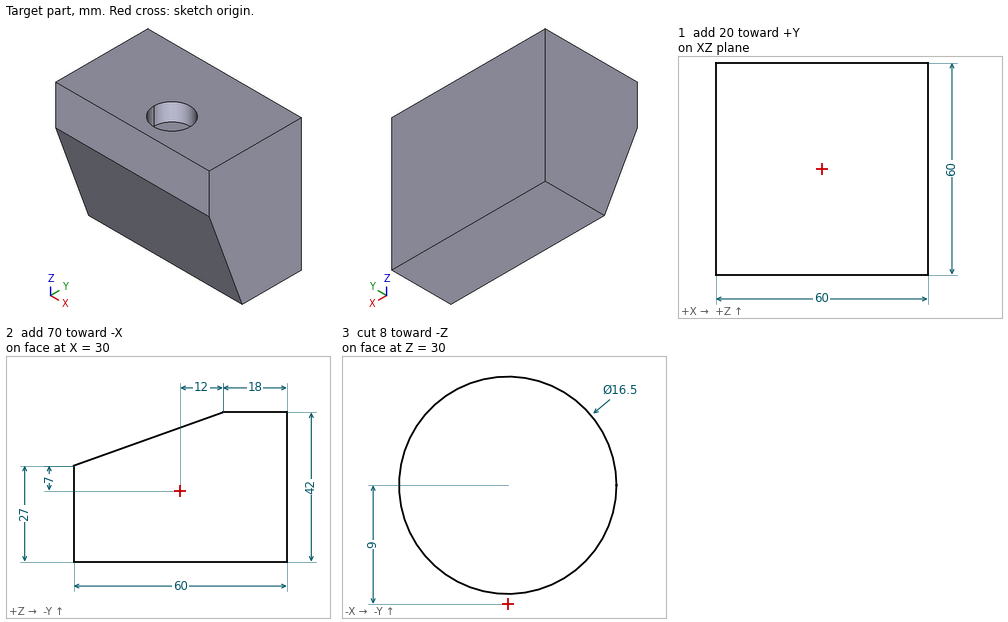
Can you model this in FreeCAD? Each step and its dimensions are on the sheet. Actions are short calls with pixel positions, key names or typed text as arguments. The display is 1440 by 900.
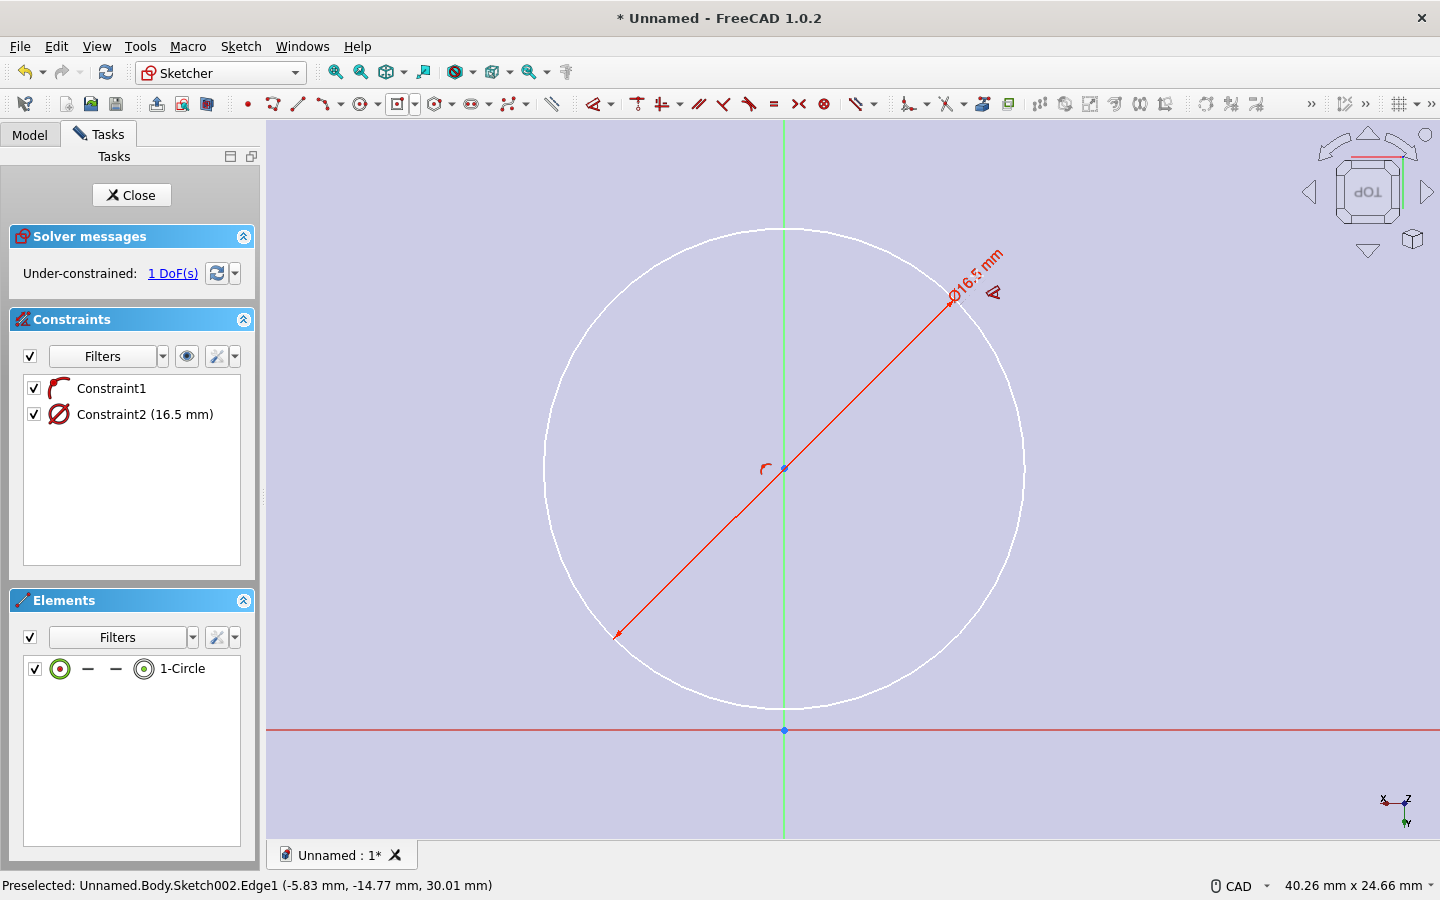
click(784, 469)
click(818, 600)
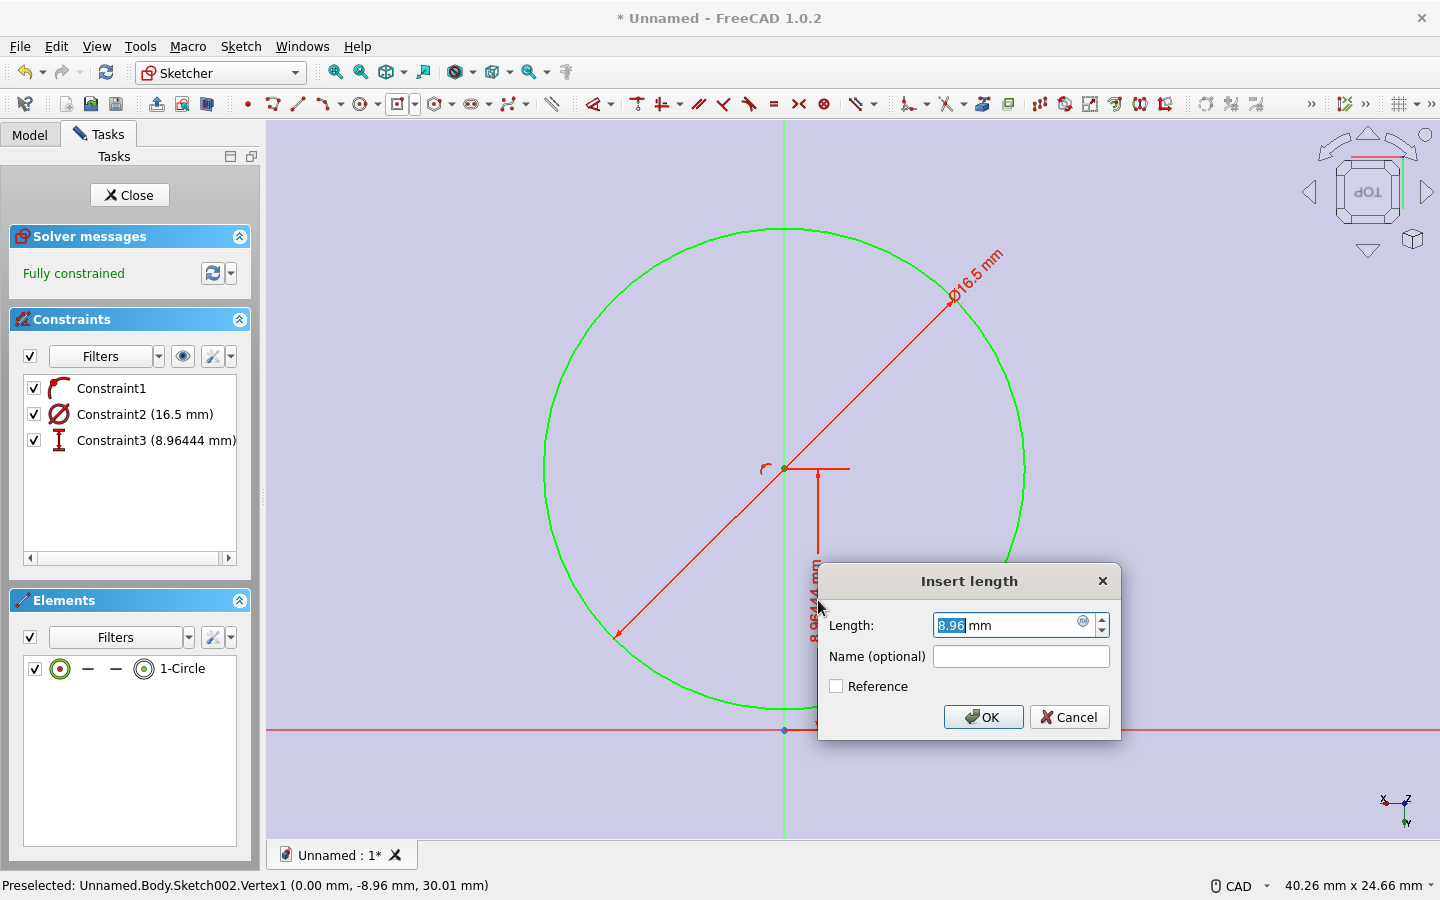
text(9)
key(Return)
key(Escape)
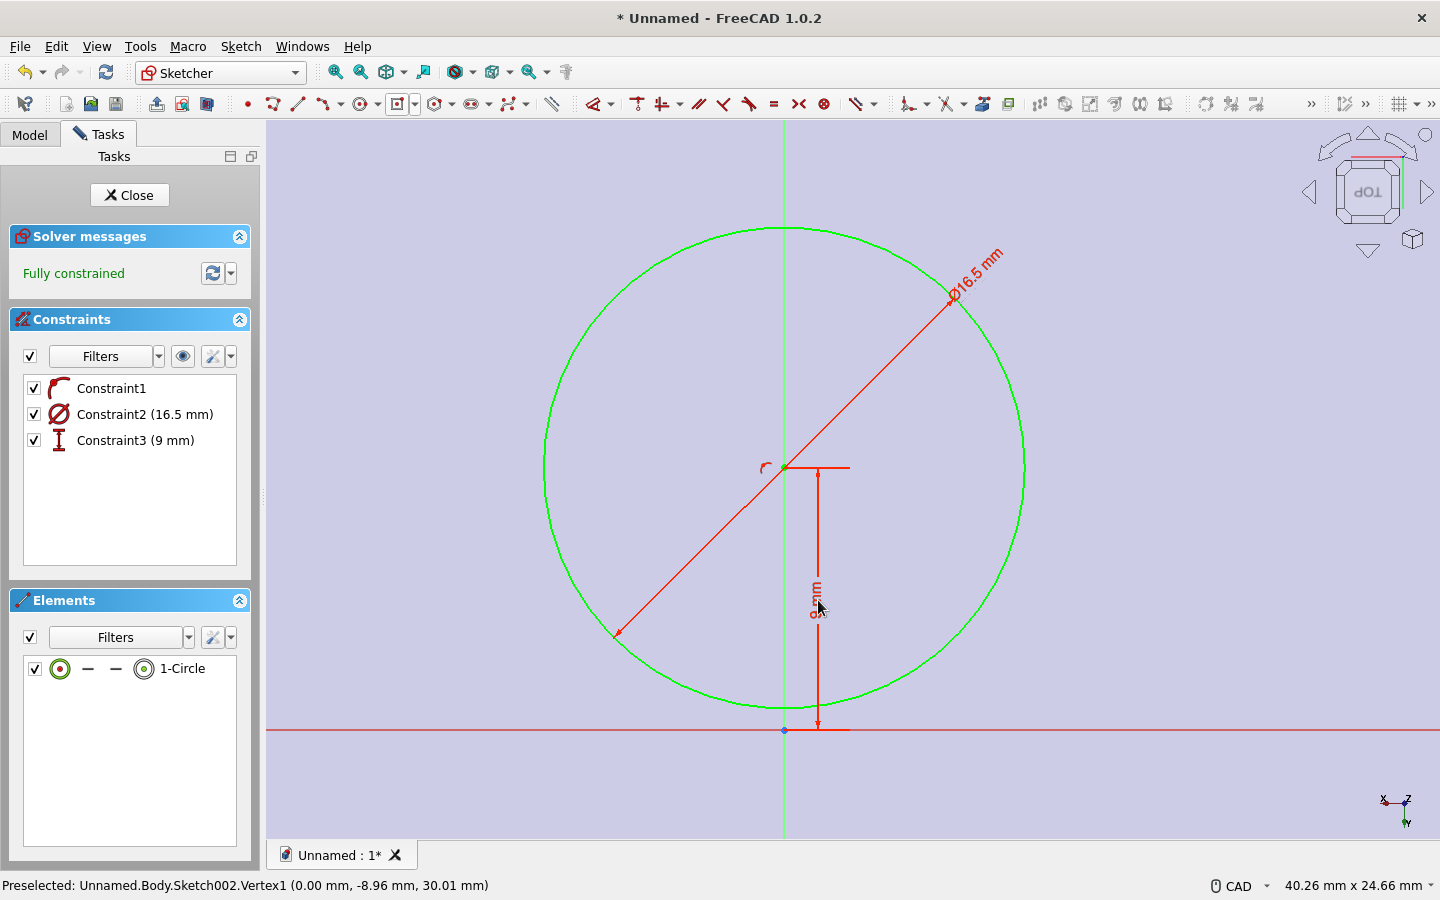
click(130, 195)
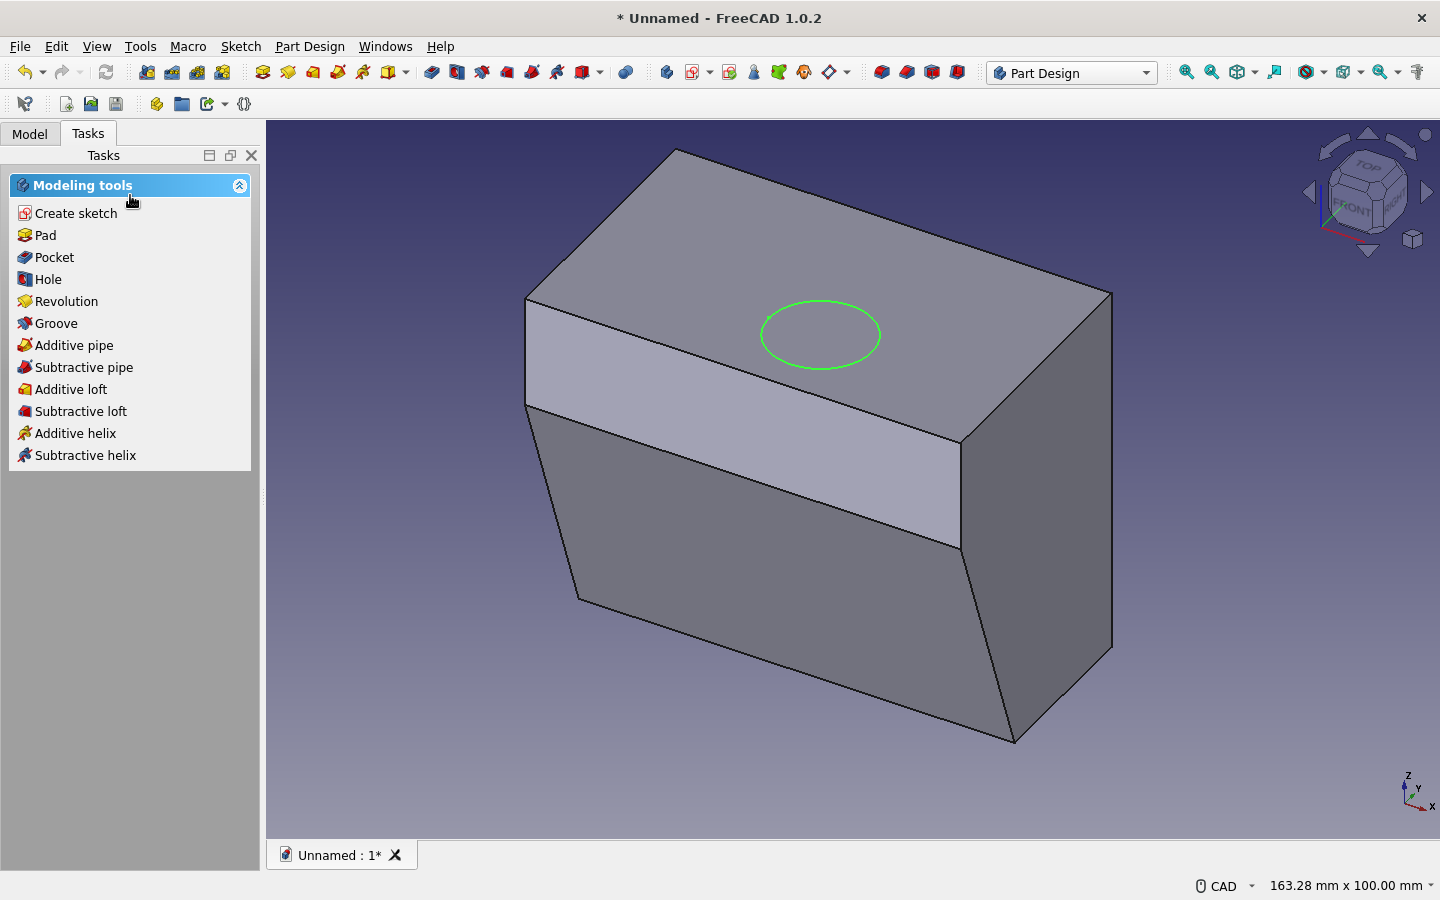
click(432, 72)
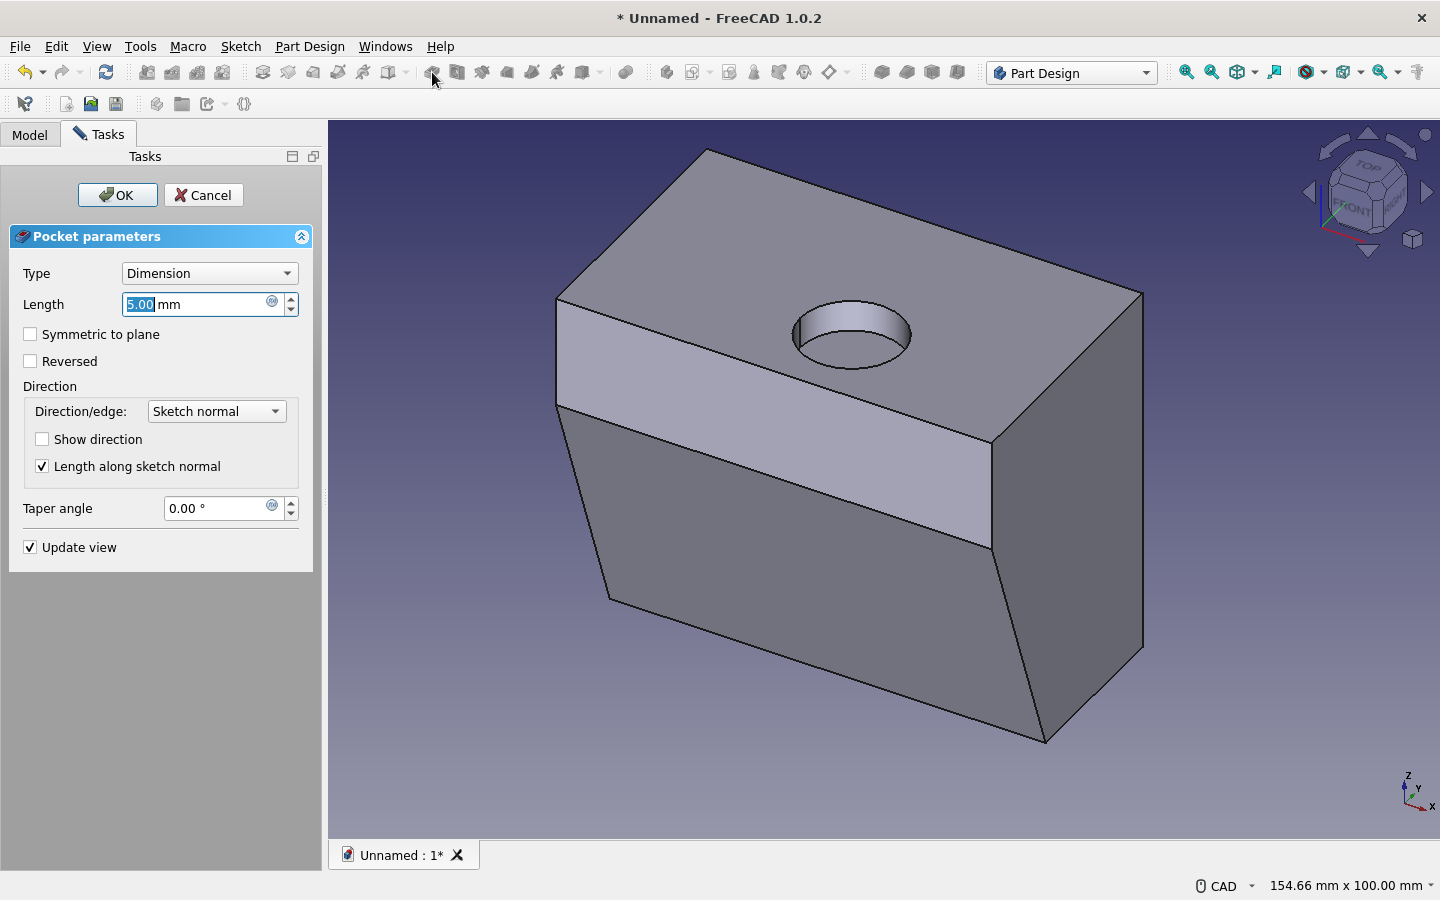
text(8)
key(Tab)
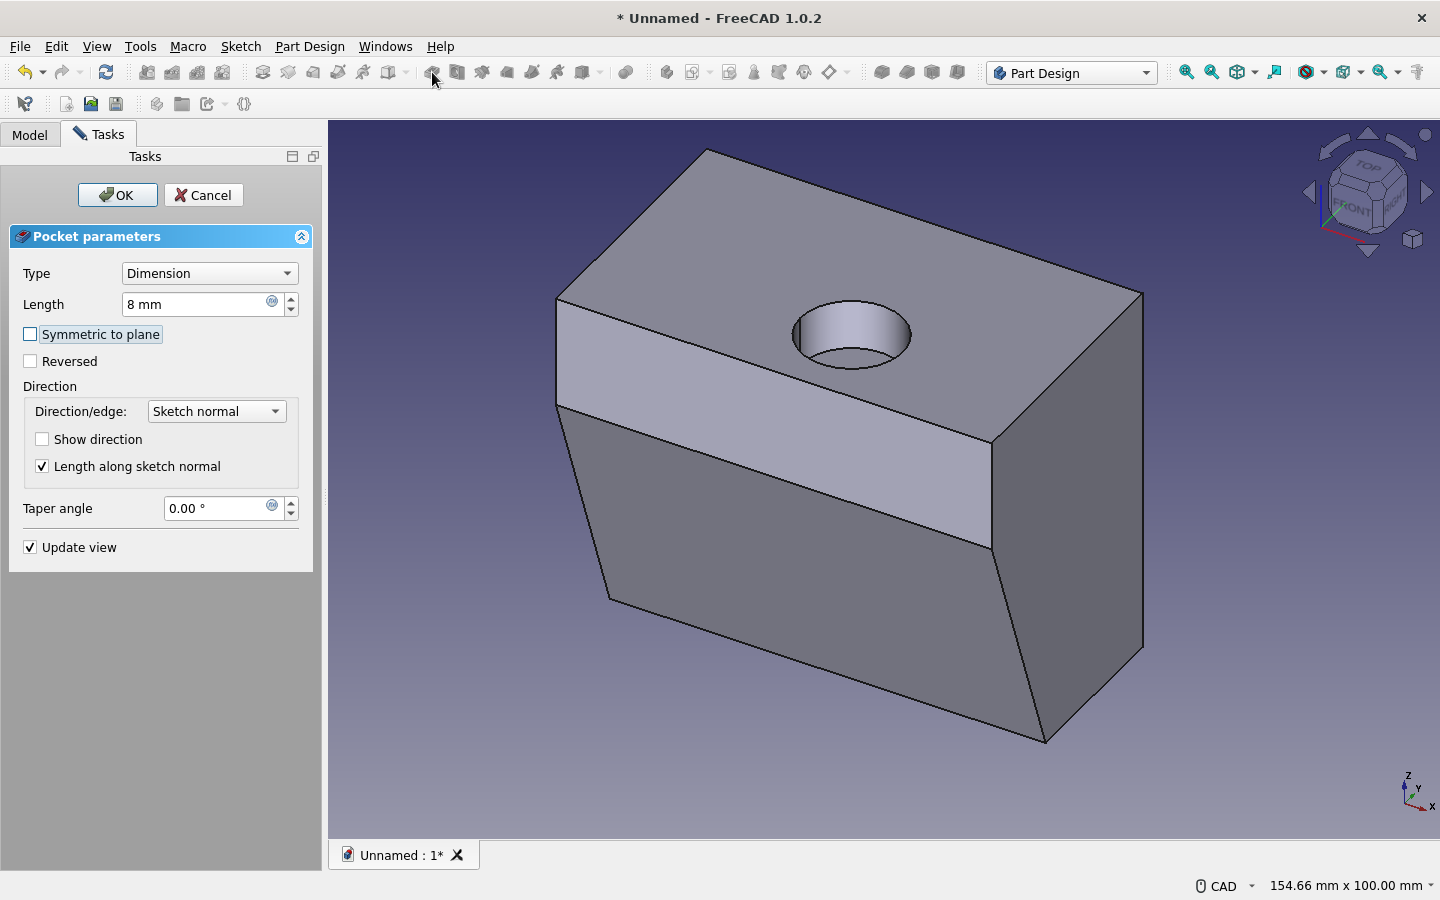
click(118, 195)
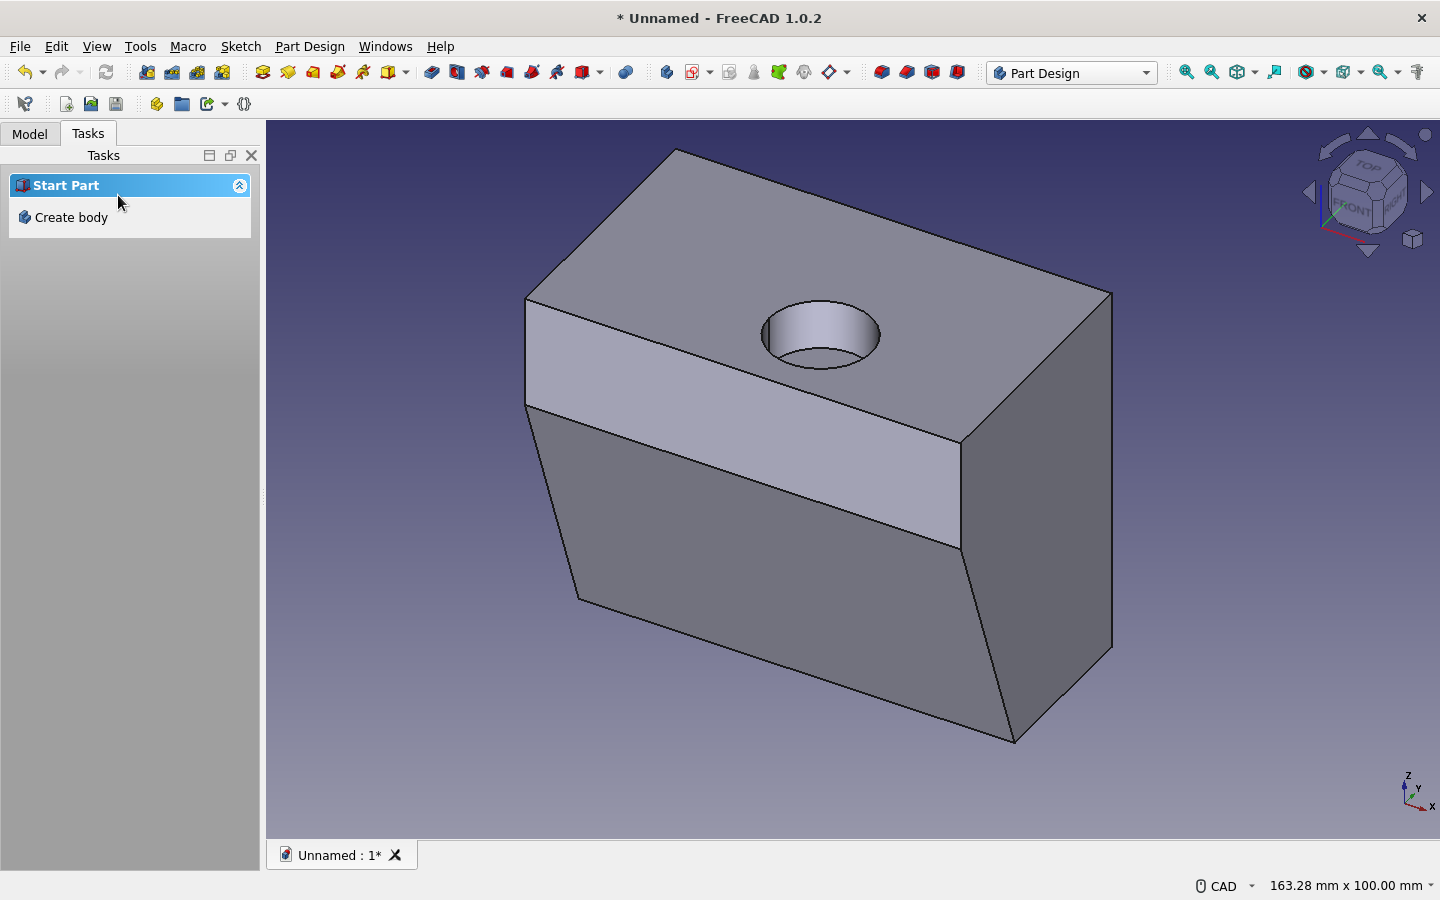
key(0)